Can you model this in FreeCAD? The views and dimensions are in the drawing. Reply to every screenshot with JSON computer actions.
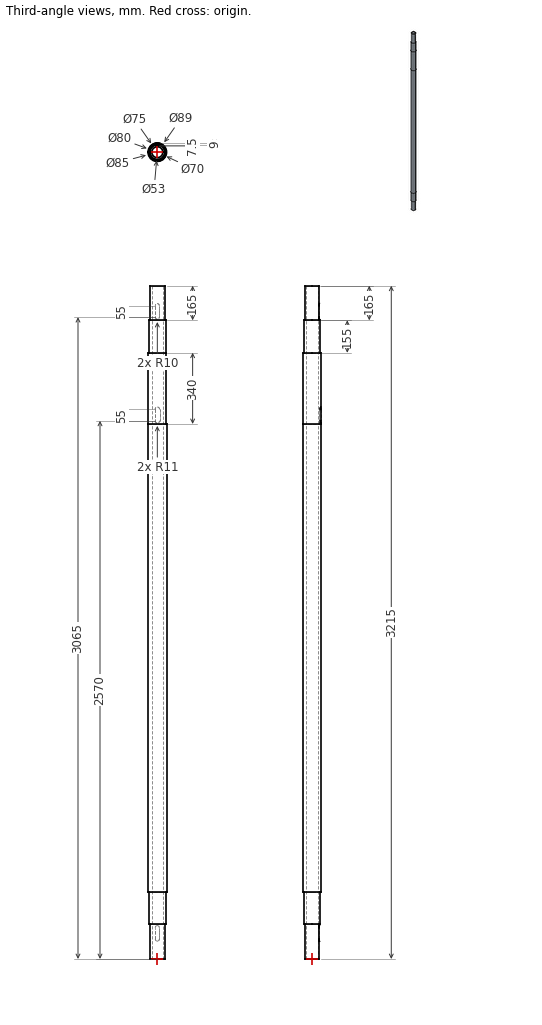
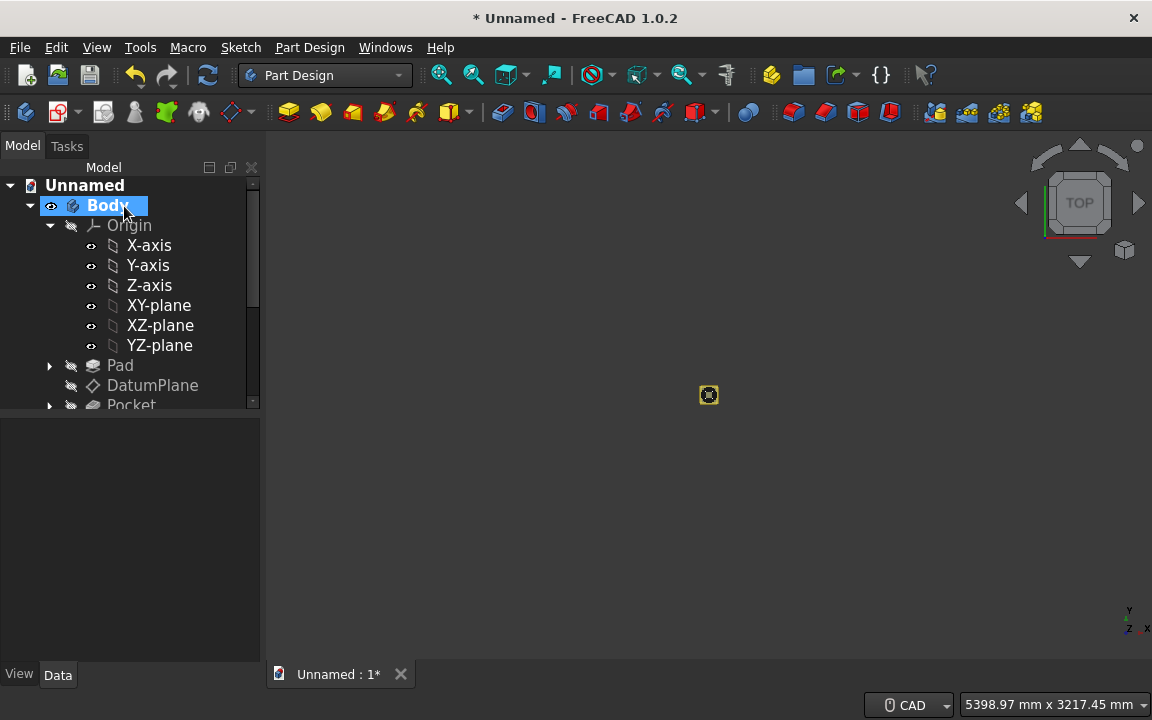
{"action": "left_click", "coordinate": [116, 406]}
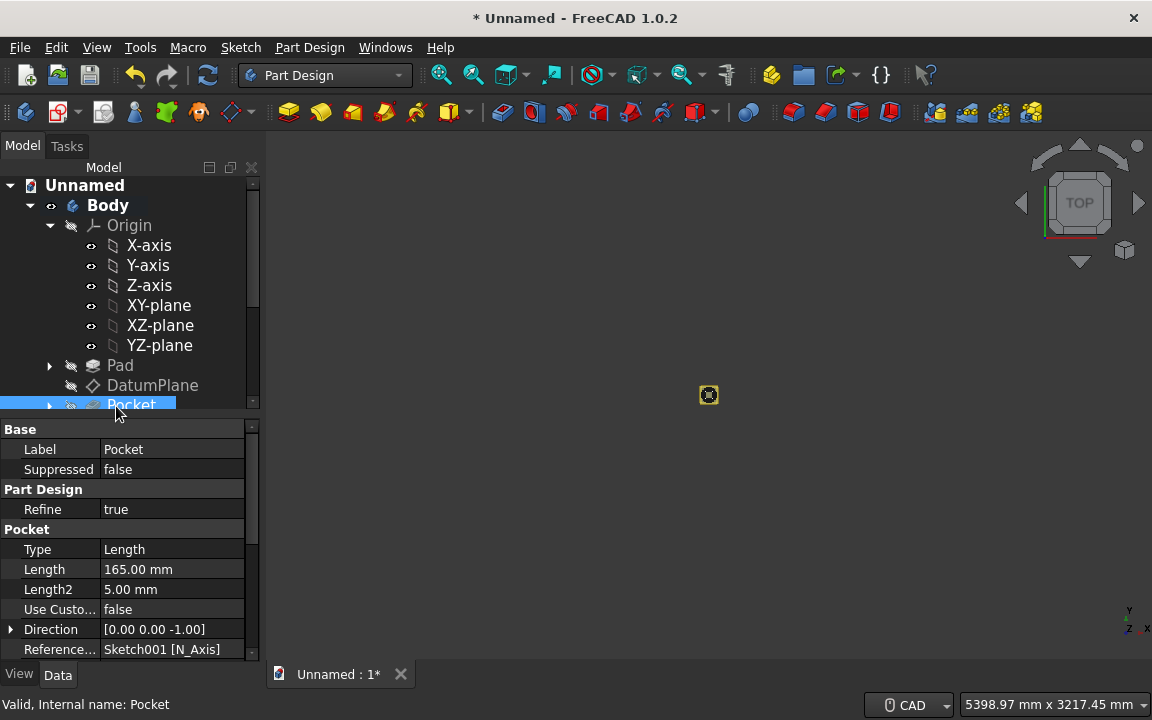
{"action": "scroll", "coordinate": [100, 301], "scroll_direction": "down", "scroll_amount": 3}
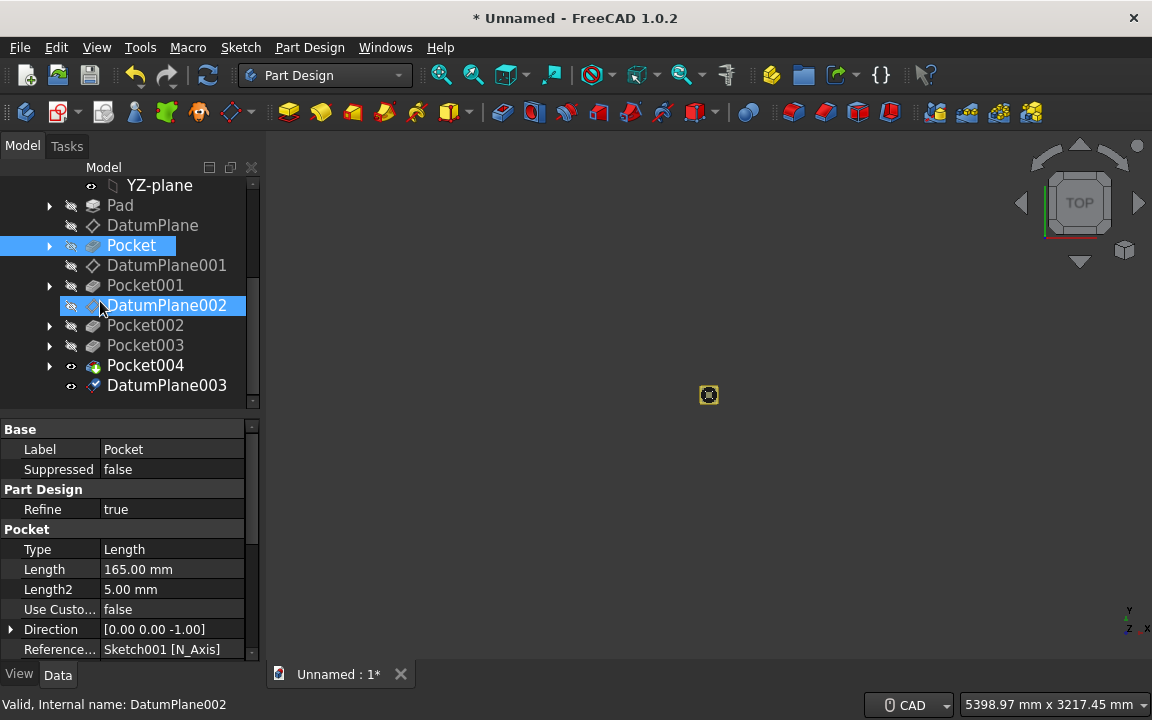
{"action": "left_click", "coordinate": [116, 286], "text": "ctrl"}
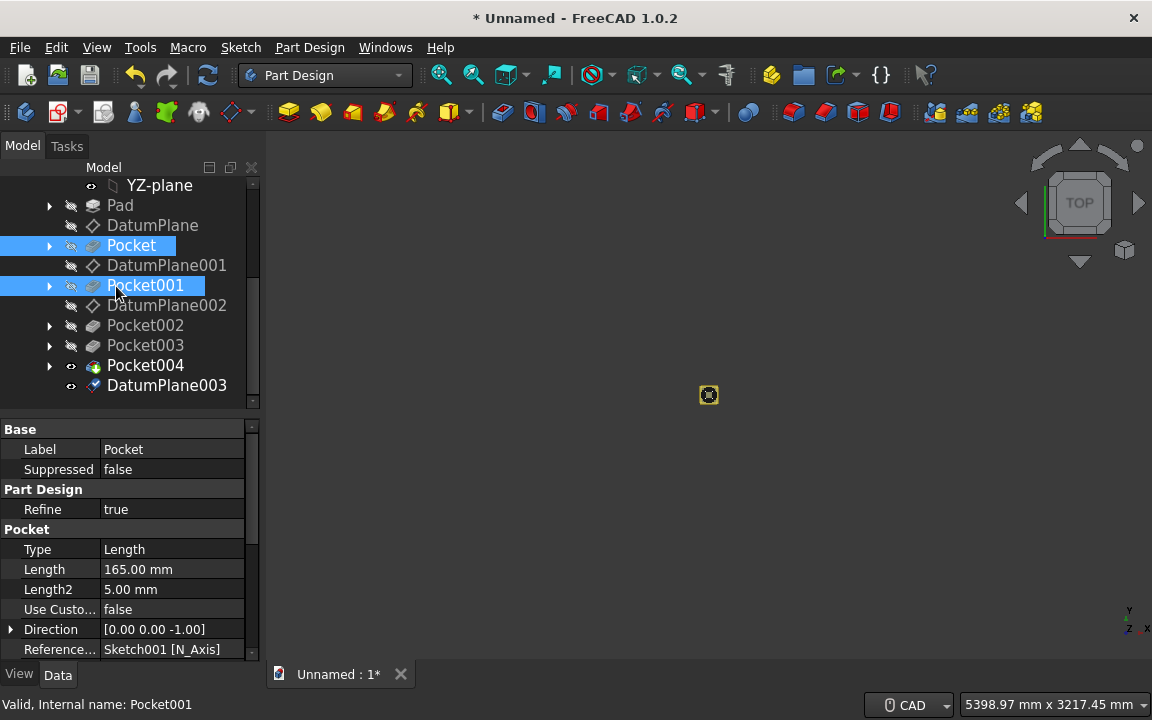
{"action": "left_click", "coordinate": [116, 366], "text": "ctrl"}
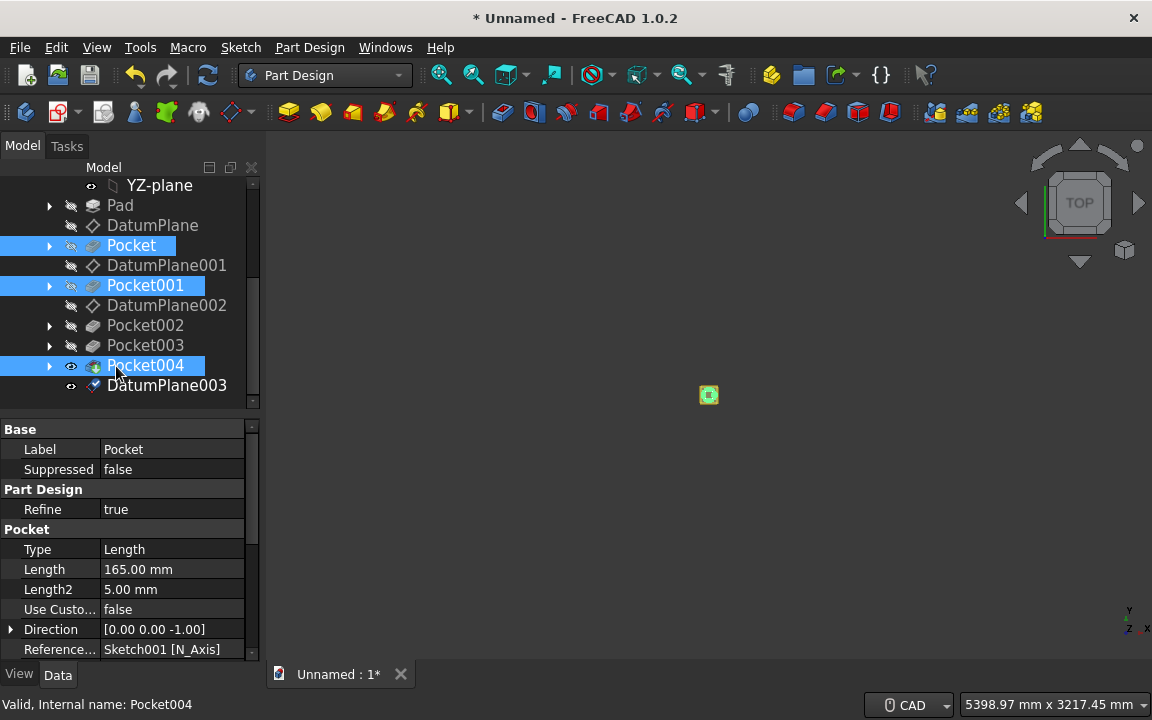
{"action": "left_click", "coordinate": [936, 112]}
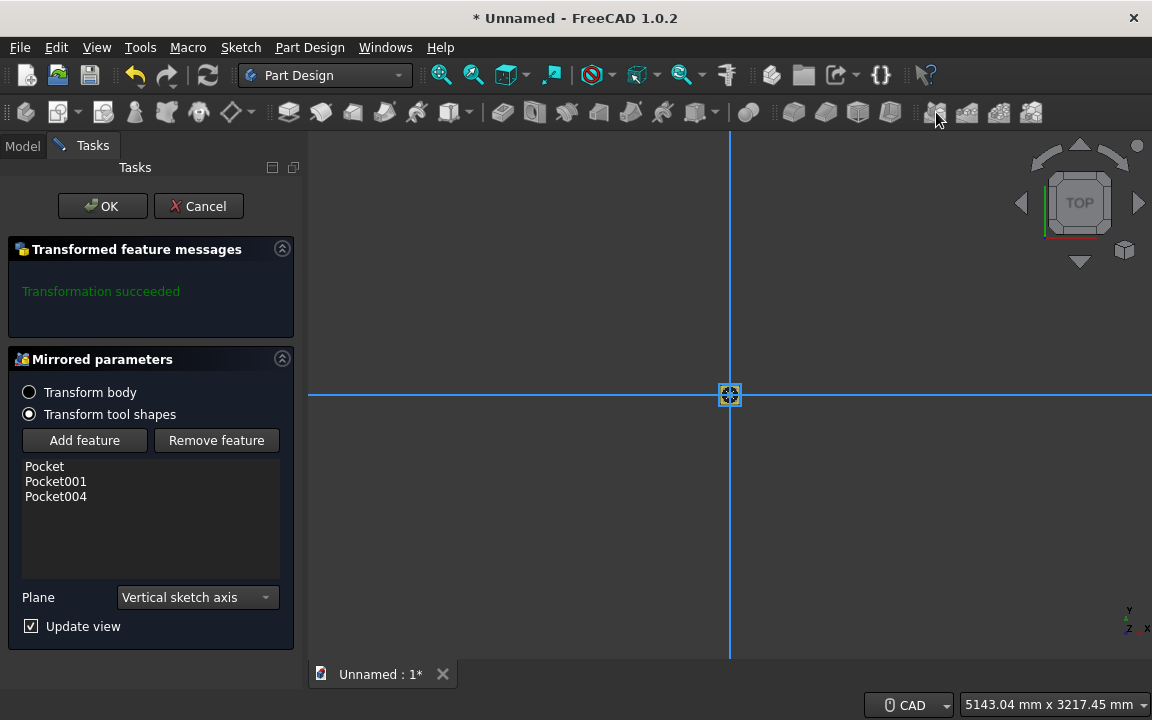
{"action": "left_click", "coordinate": [198, 598]}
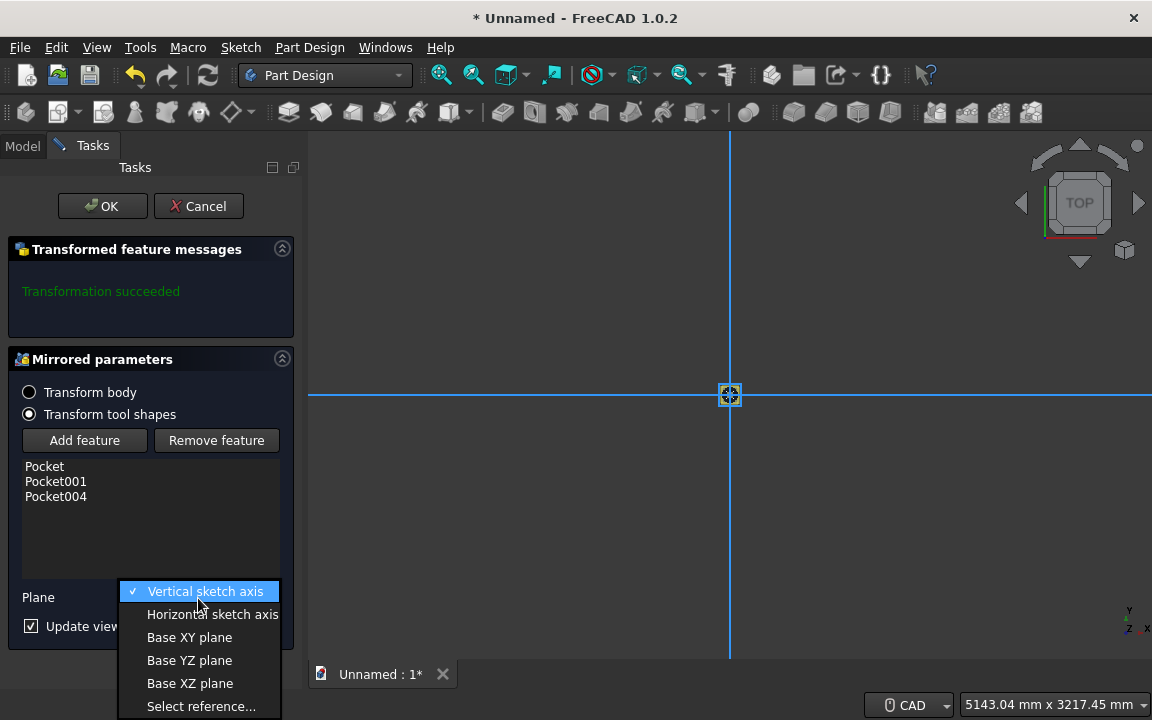
{"action": "left_click", "coordinate": [198, 706]}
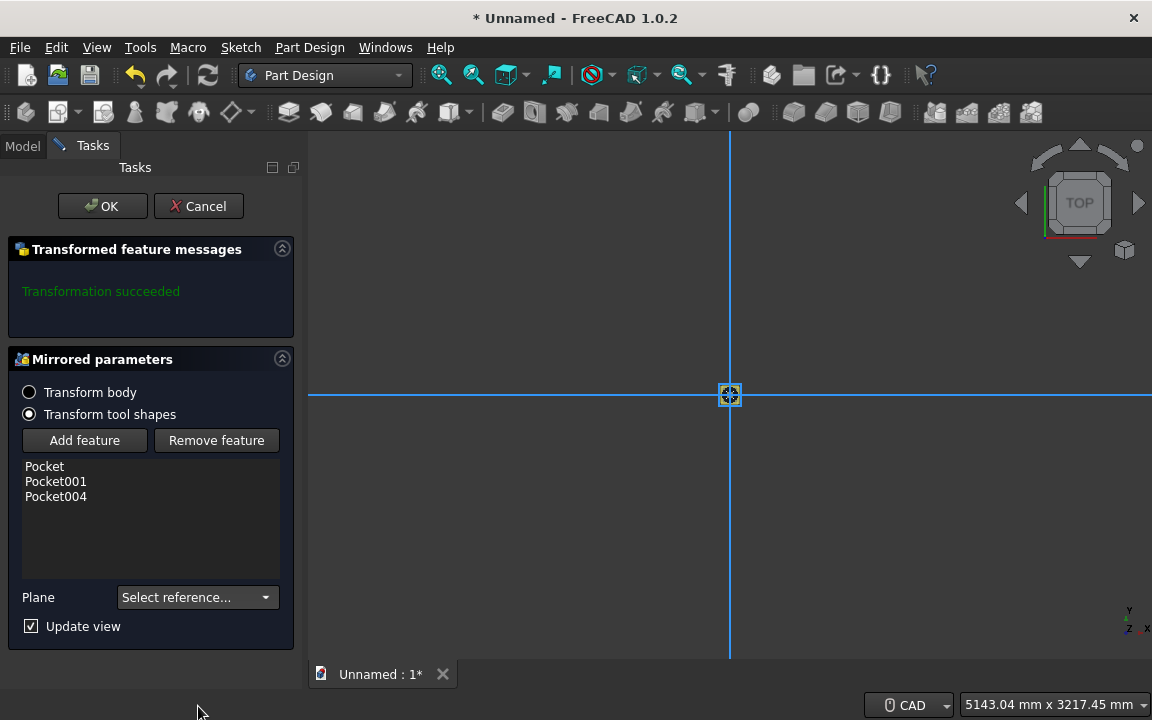
{"action": "left_click", "coordinate": [23, 145]}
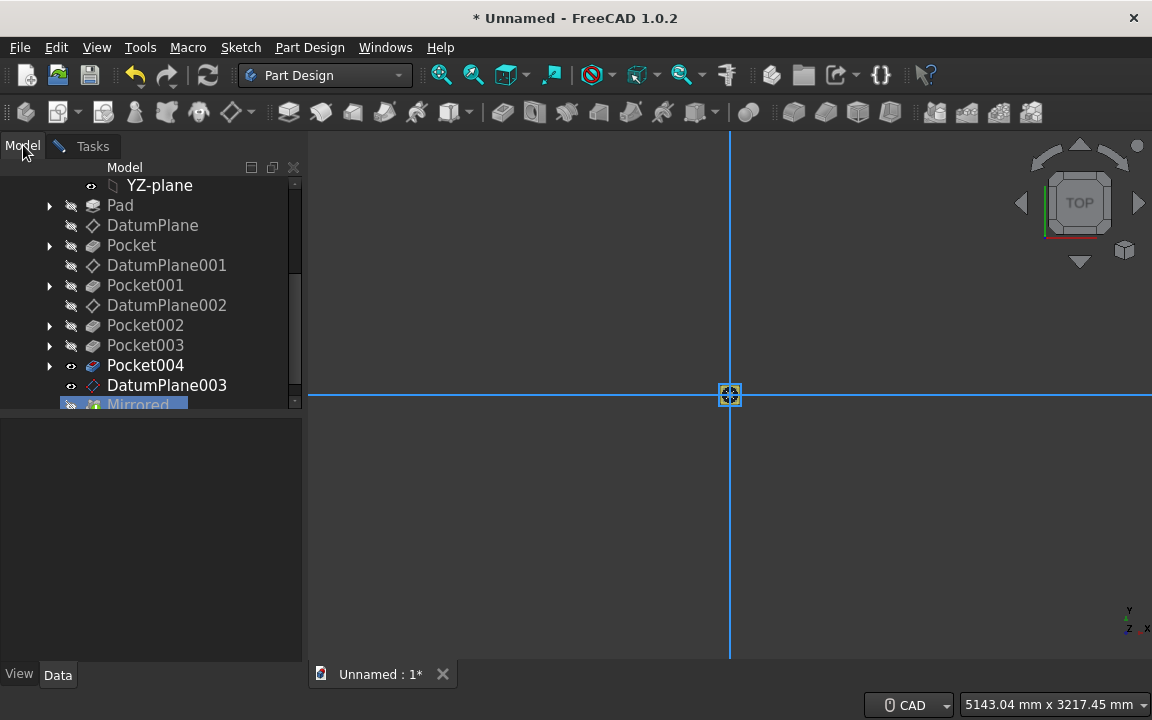
{"action": "left_click", "coordinate": [116, 386]}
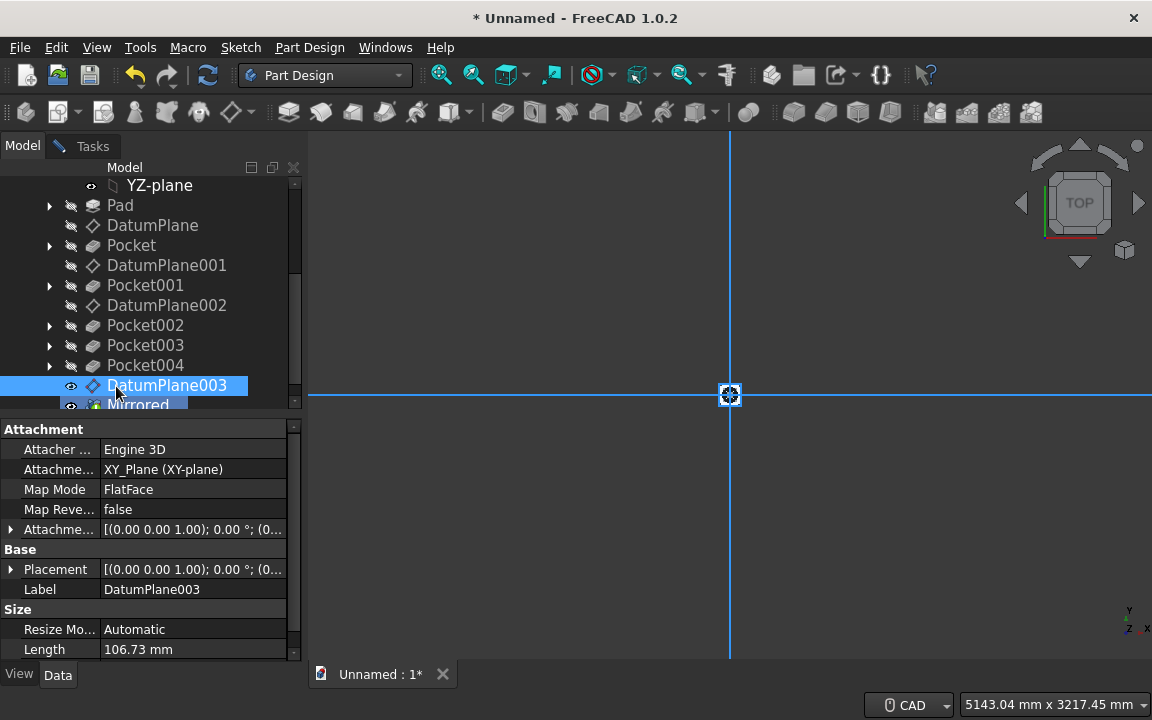
{"action": "left_click", "coordinate": [84, 145]}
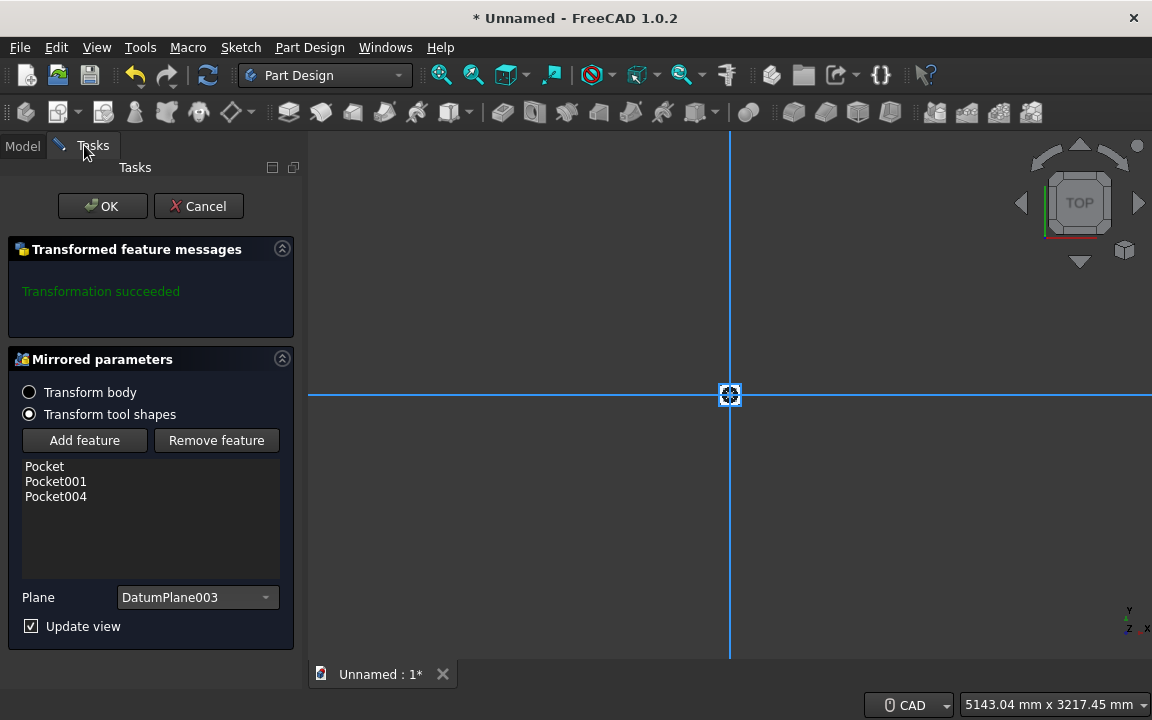
{"action": "left_click", "coordinate": [103, 206]}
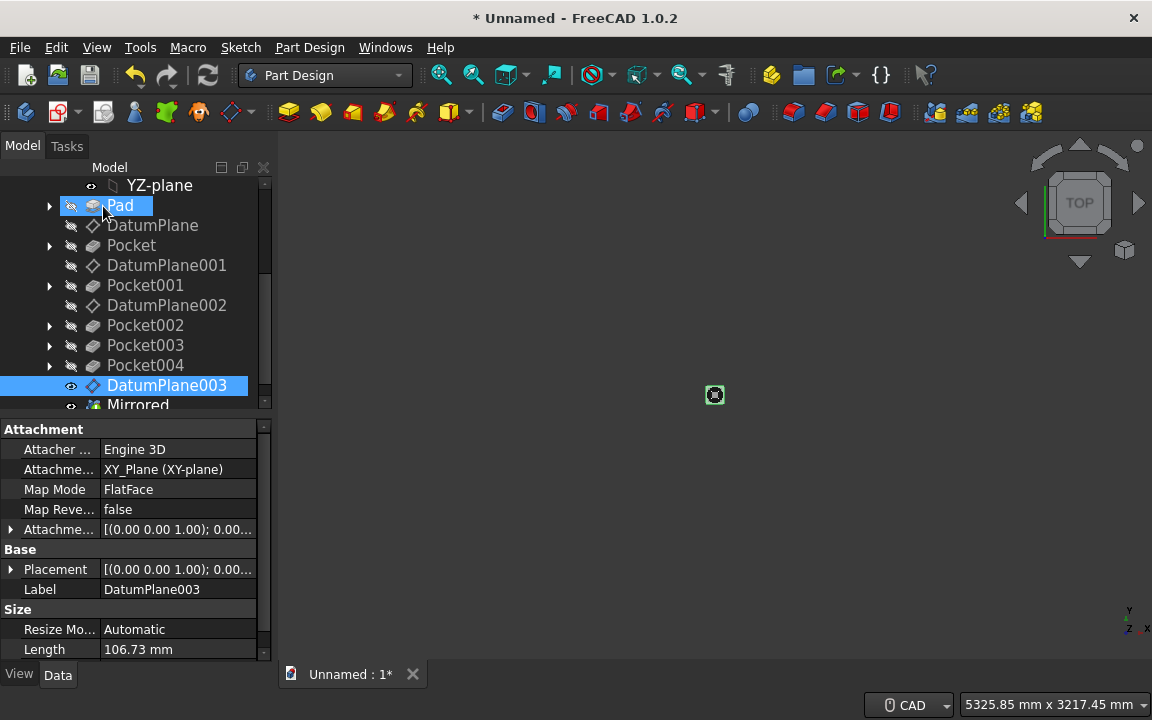
{"action": "left_click", "coordinate": [116, 386]}
{"action": "key", "text": "space"}